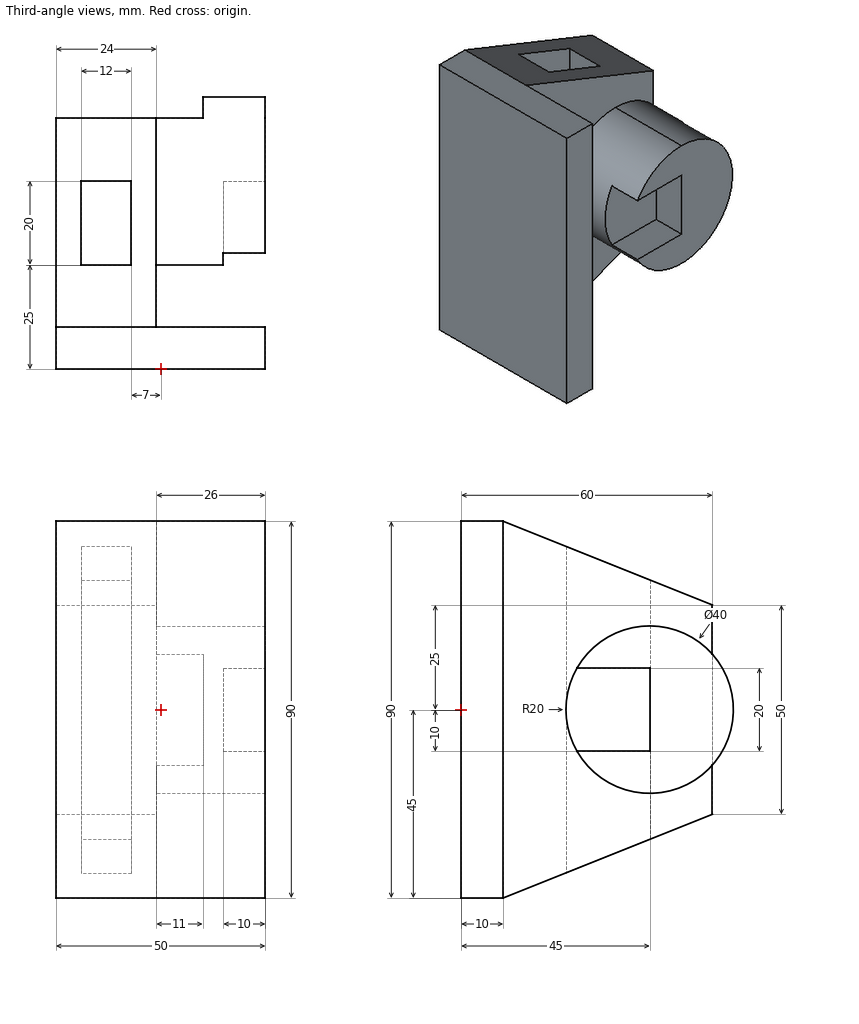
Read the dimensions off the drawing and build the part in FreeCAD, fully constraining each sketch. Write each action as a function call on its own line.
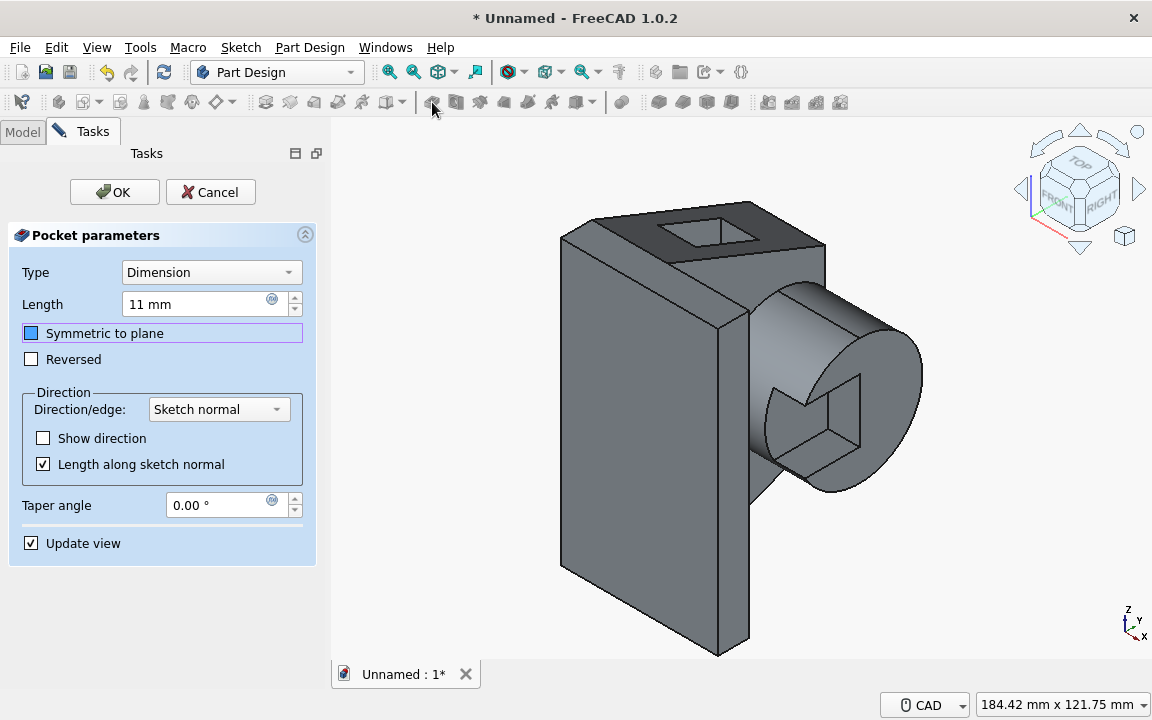
click(30, 359)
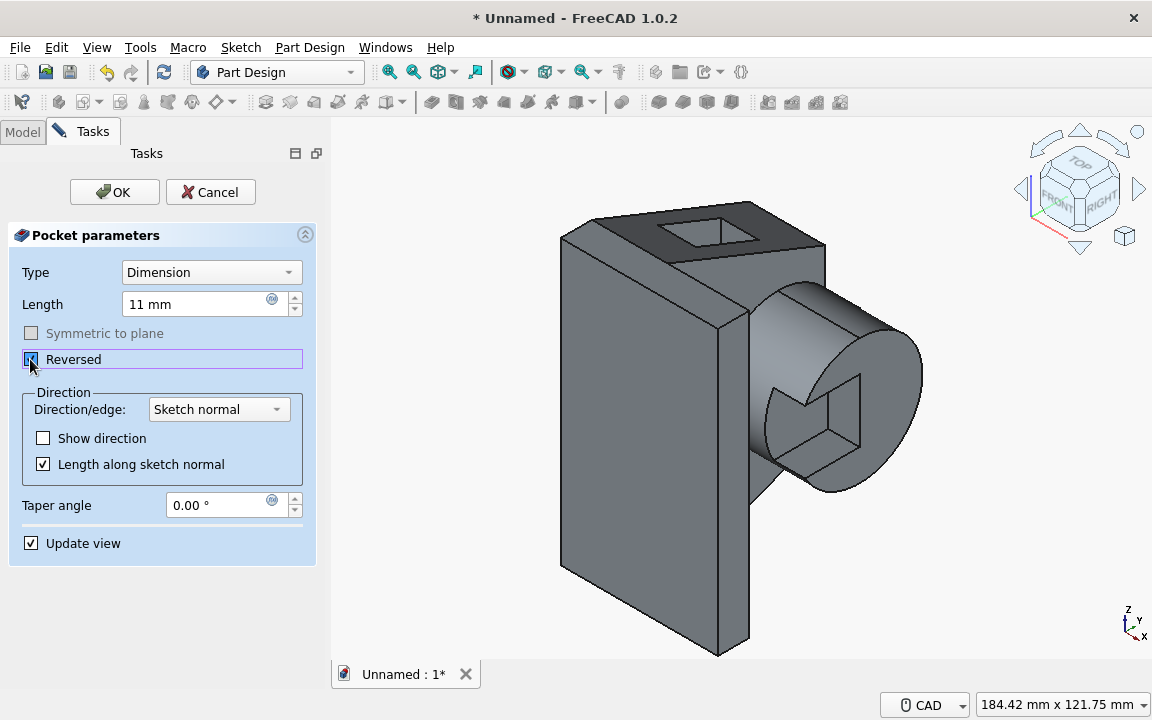
click(115, 192)